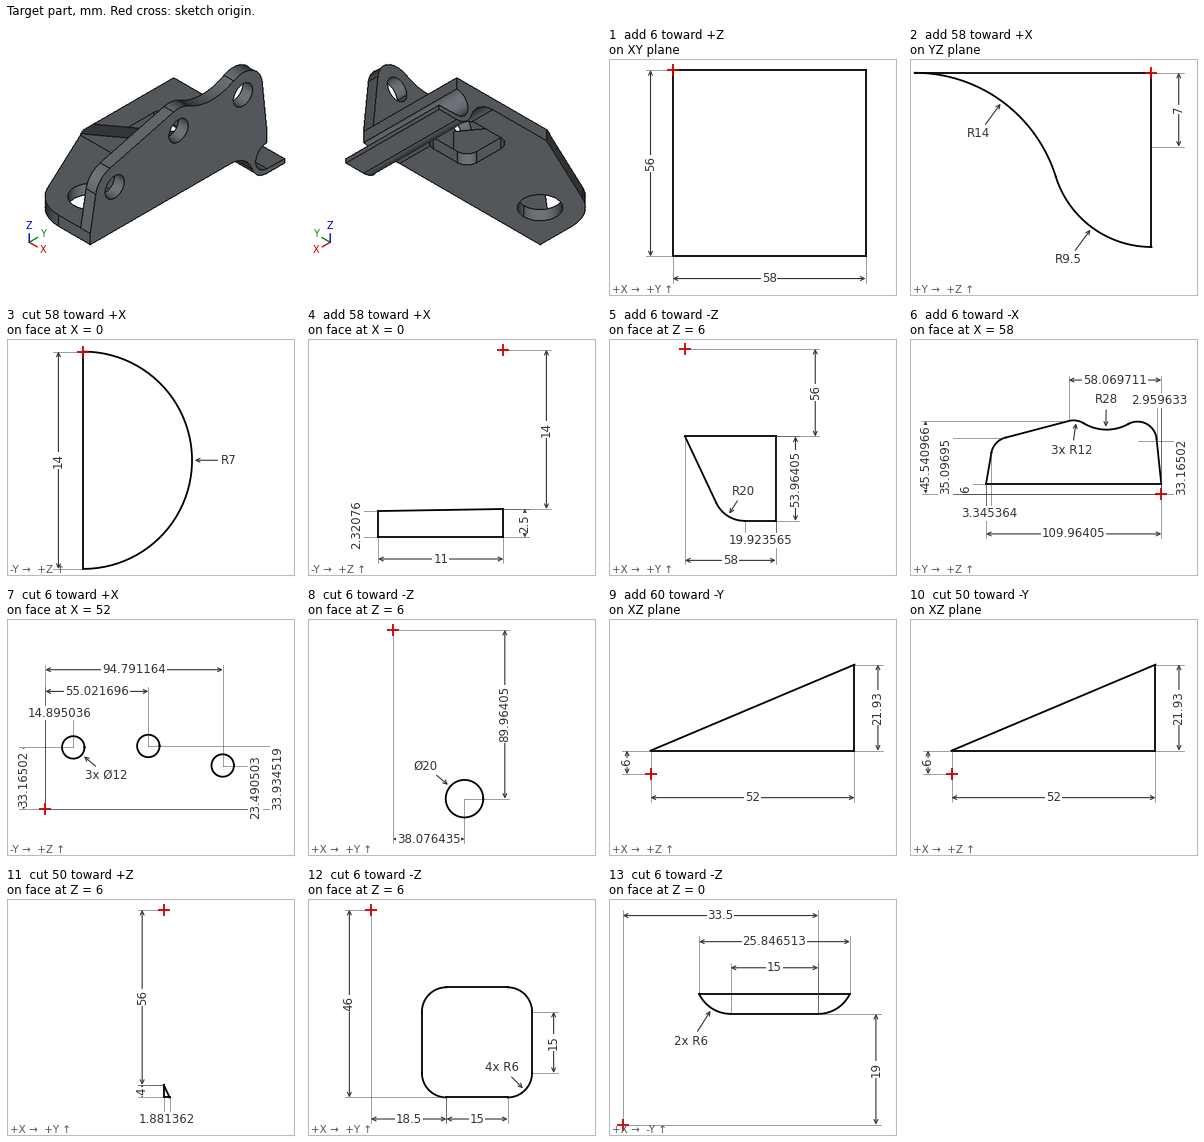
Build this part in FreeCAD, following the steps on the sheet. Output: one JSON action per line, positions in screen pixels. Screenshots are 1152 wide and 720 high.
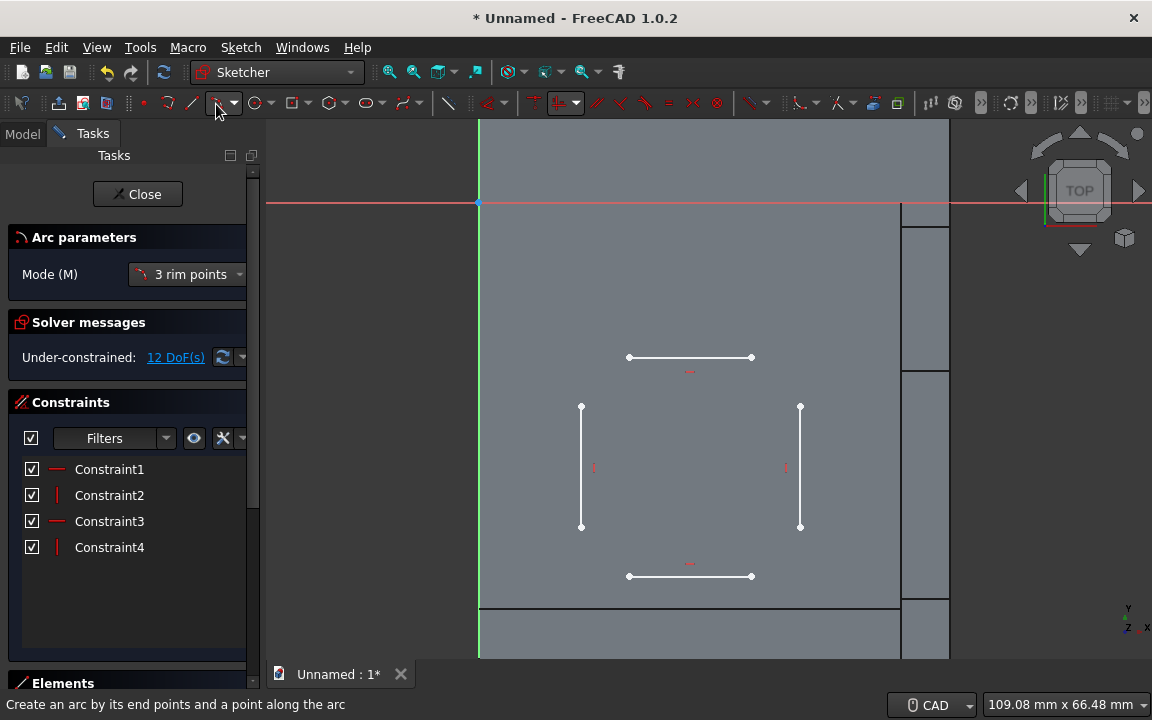
{"action": "left_click", "coordinate": [751, 577]}
{"action": "left_click", "coordinate": [800, 528]}
{"action": "left_click", "coordinate": [786, 562]}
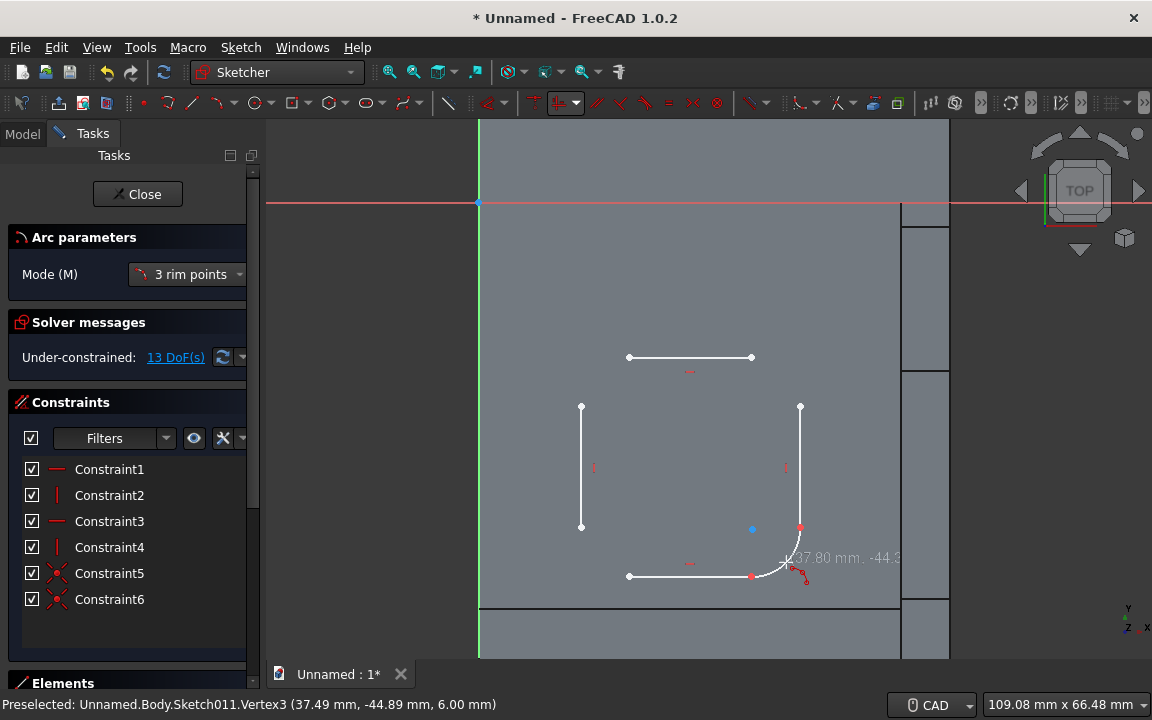
{"action": "left_click", "coordinate": [800, 407]}
{"action": "left_click", "coordinate": [751, 358]}
{"action": "left_click", "coordinate": [786, 371]}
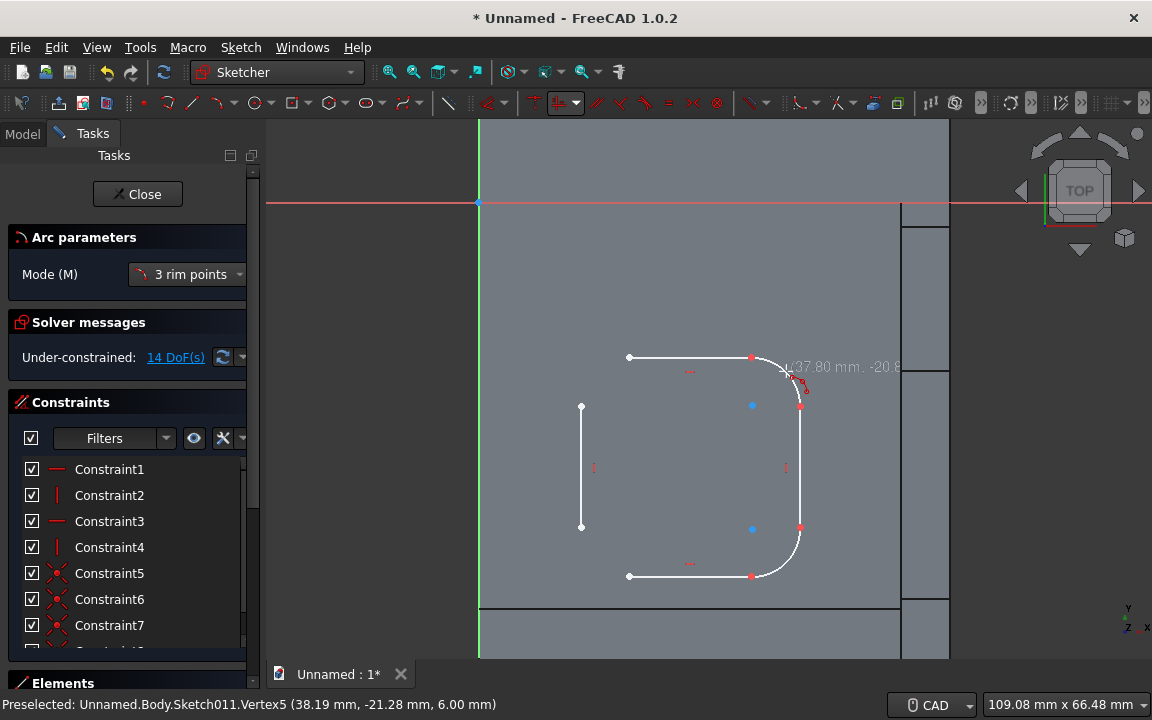
{"action": "left_click", "coordinate": [629, 358]}
{"action": "left_click", "coordinate": [581, 407]}
{"action": "left_click", "coordinate": [595, 371]}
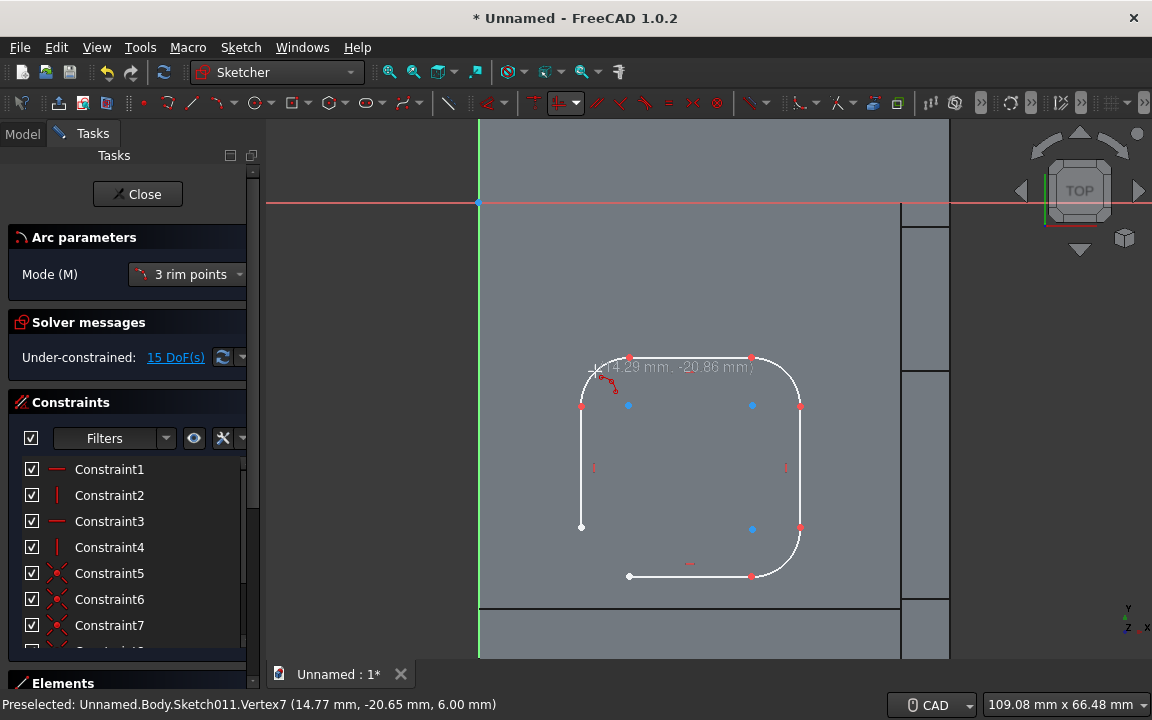
{"action": "left_click", "coordinate": [581, 528]}
{"action": "left_click", "coordinate": [629, 577]}
{"action": "left_click", "coordinate": [595, 562]}
{"action": "key", "text": "Escape"}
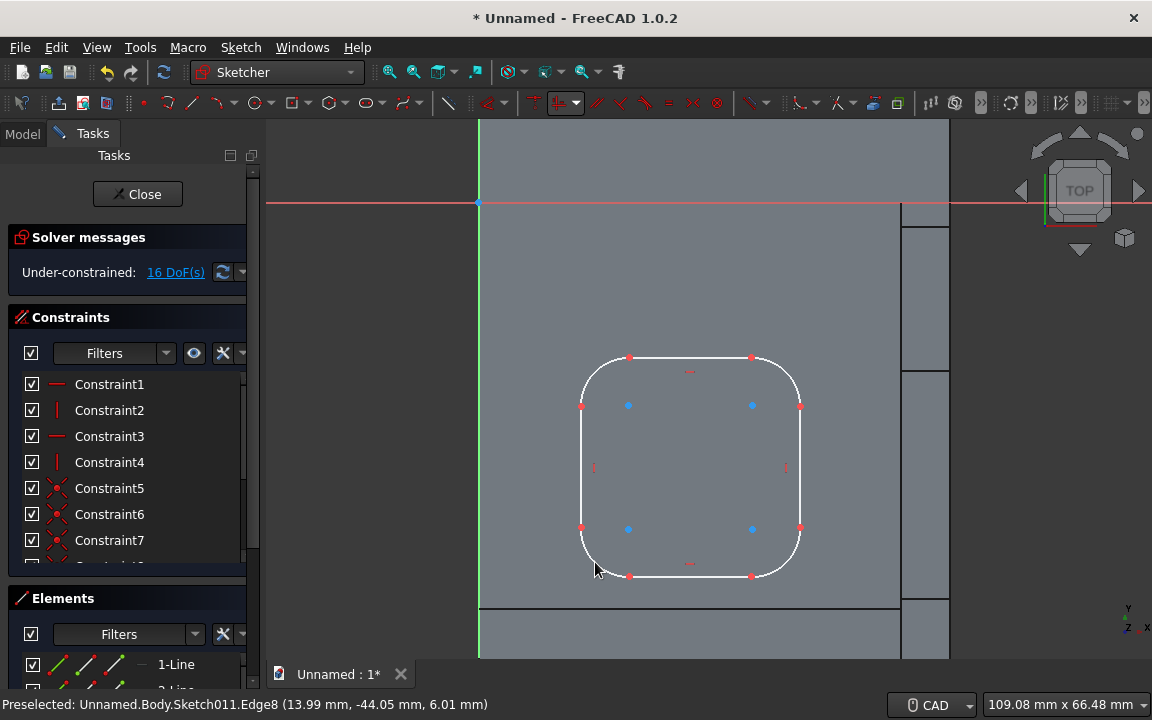
{"action": "left_click", "coordinate": [666, 577]}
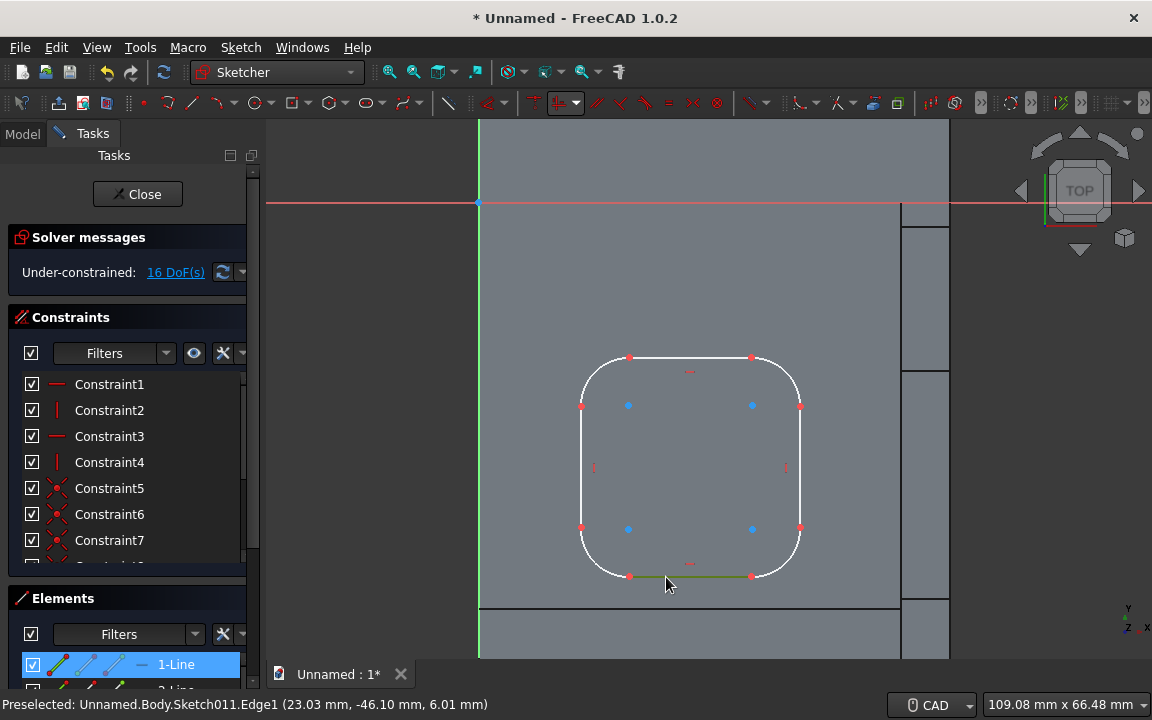
{"action": "left_click", "coordinate": [773, 572]}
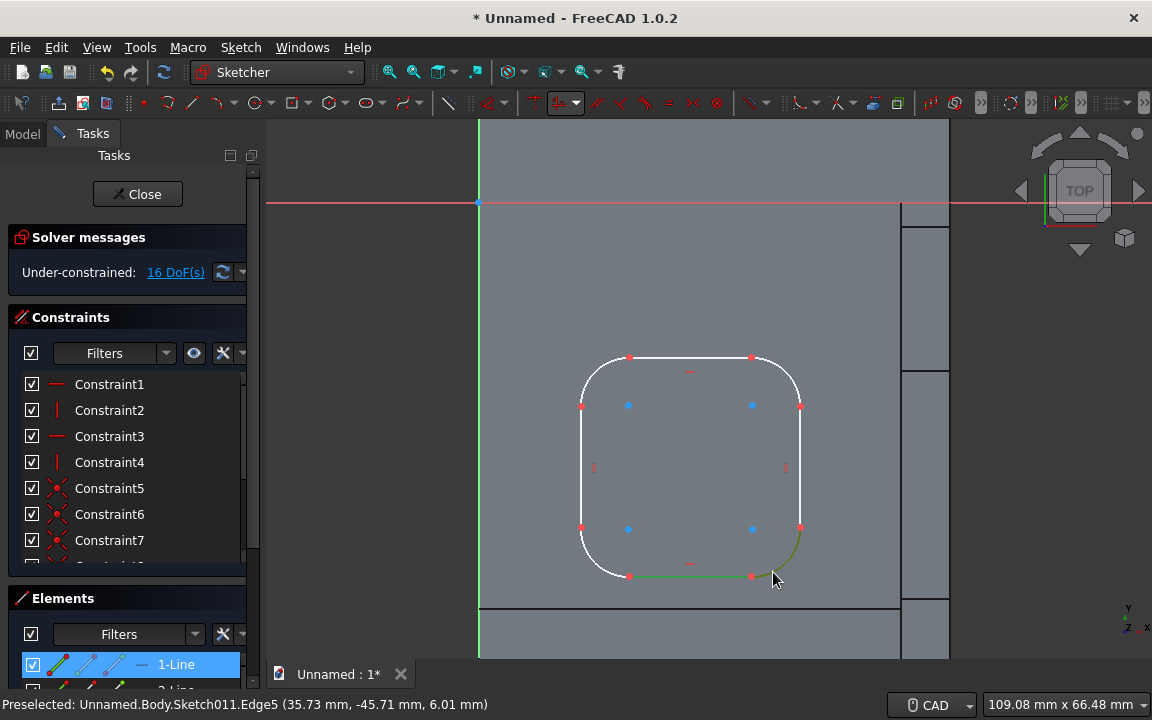
{"action": "left_click", "coordinate": [646, 104]}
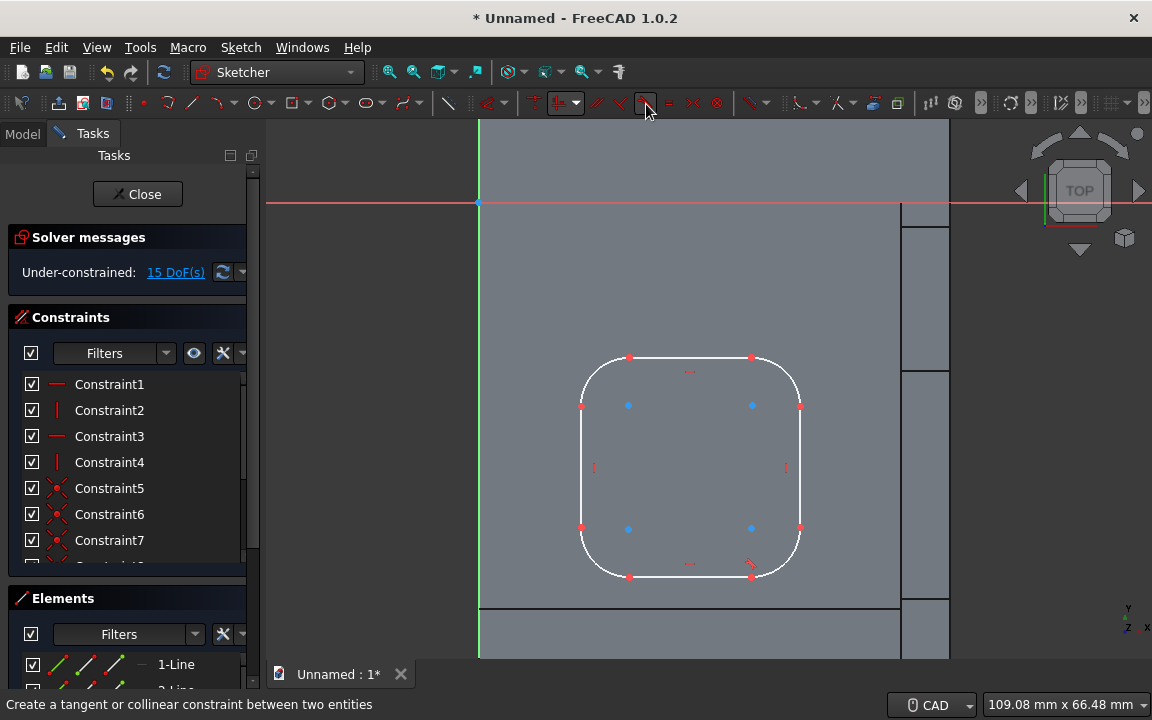
{"action": "left_click", "coordinate": [666, 577]}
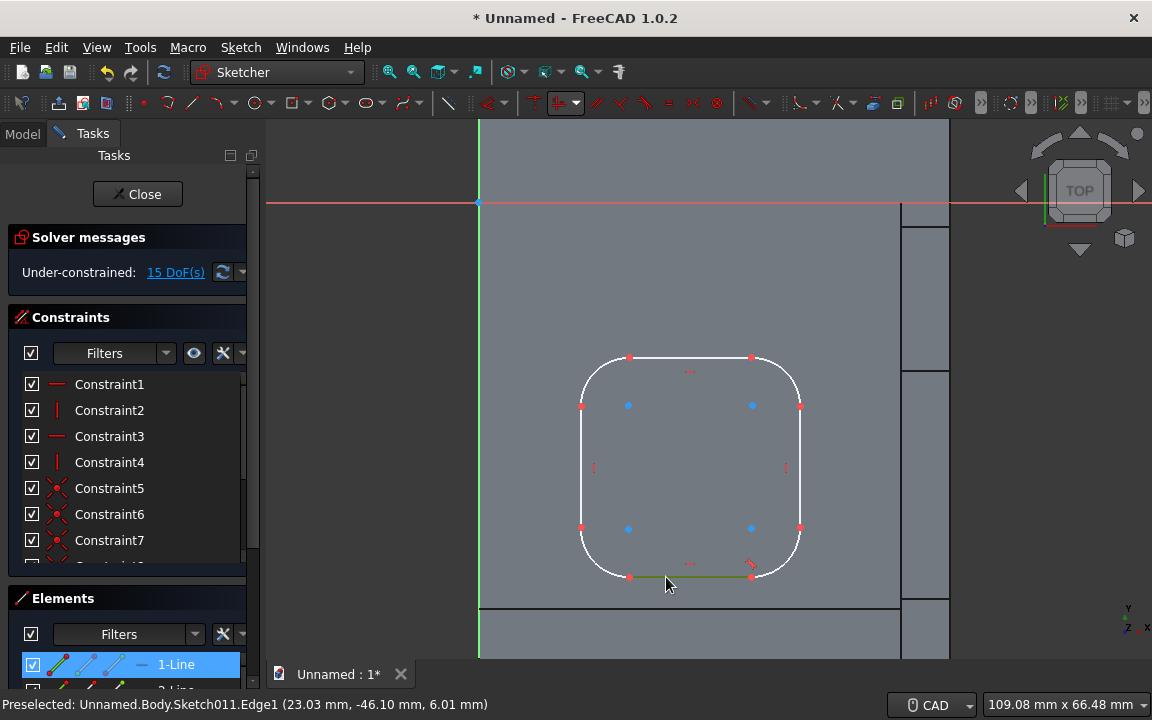
{"action": "left_click", "coordinate": [586, 550]}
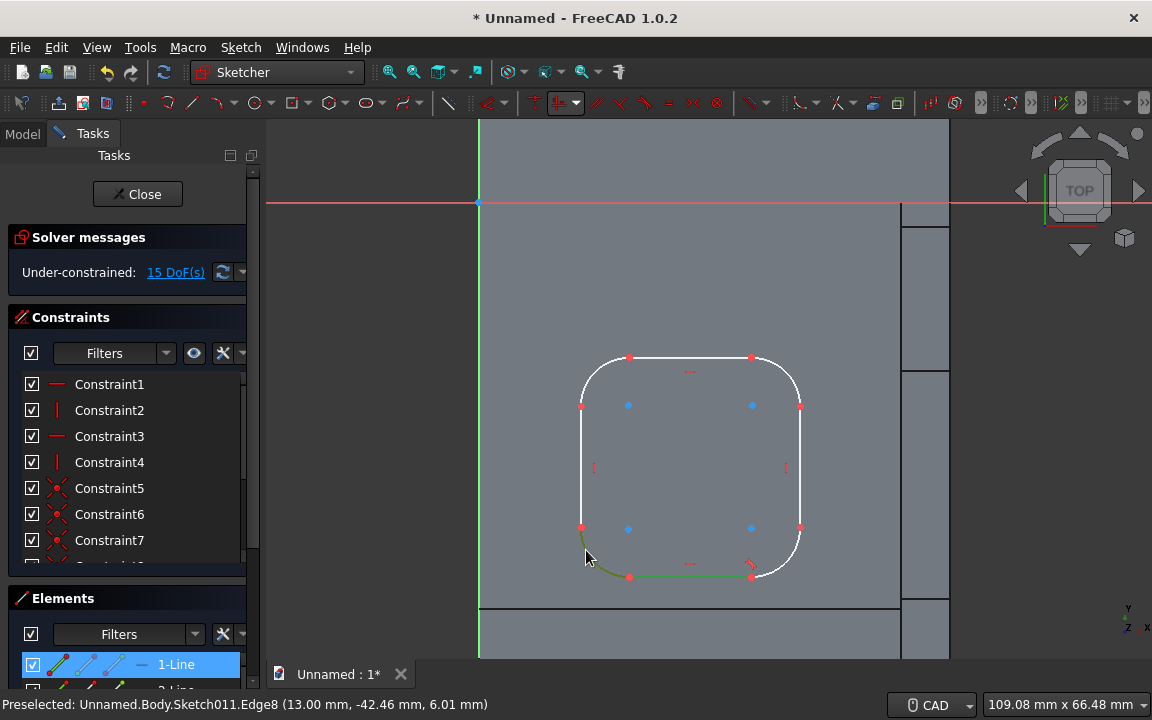
{"action": "key", "text": "t"}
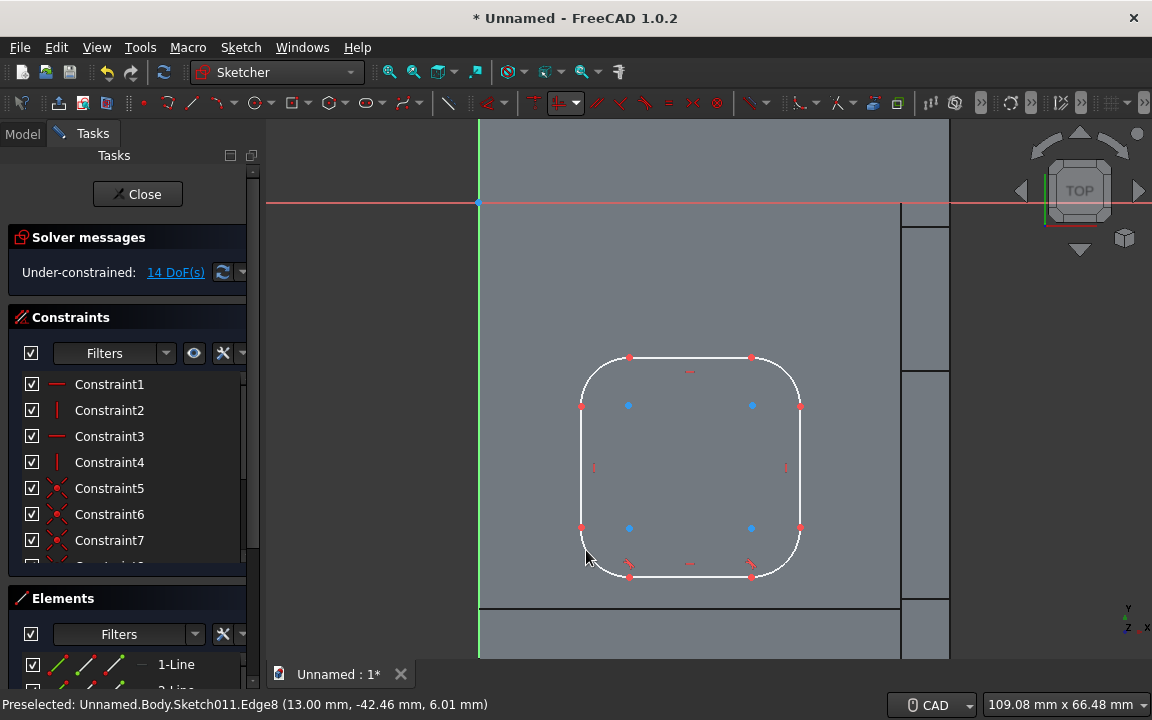
{"action": "left_click", "coordinate": [800, 492]}